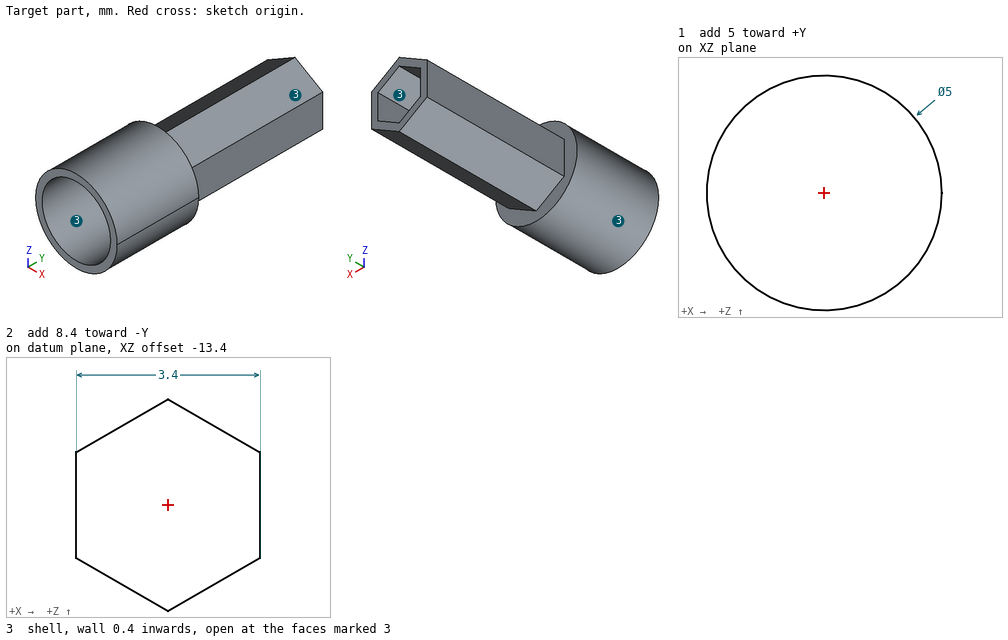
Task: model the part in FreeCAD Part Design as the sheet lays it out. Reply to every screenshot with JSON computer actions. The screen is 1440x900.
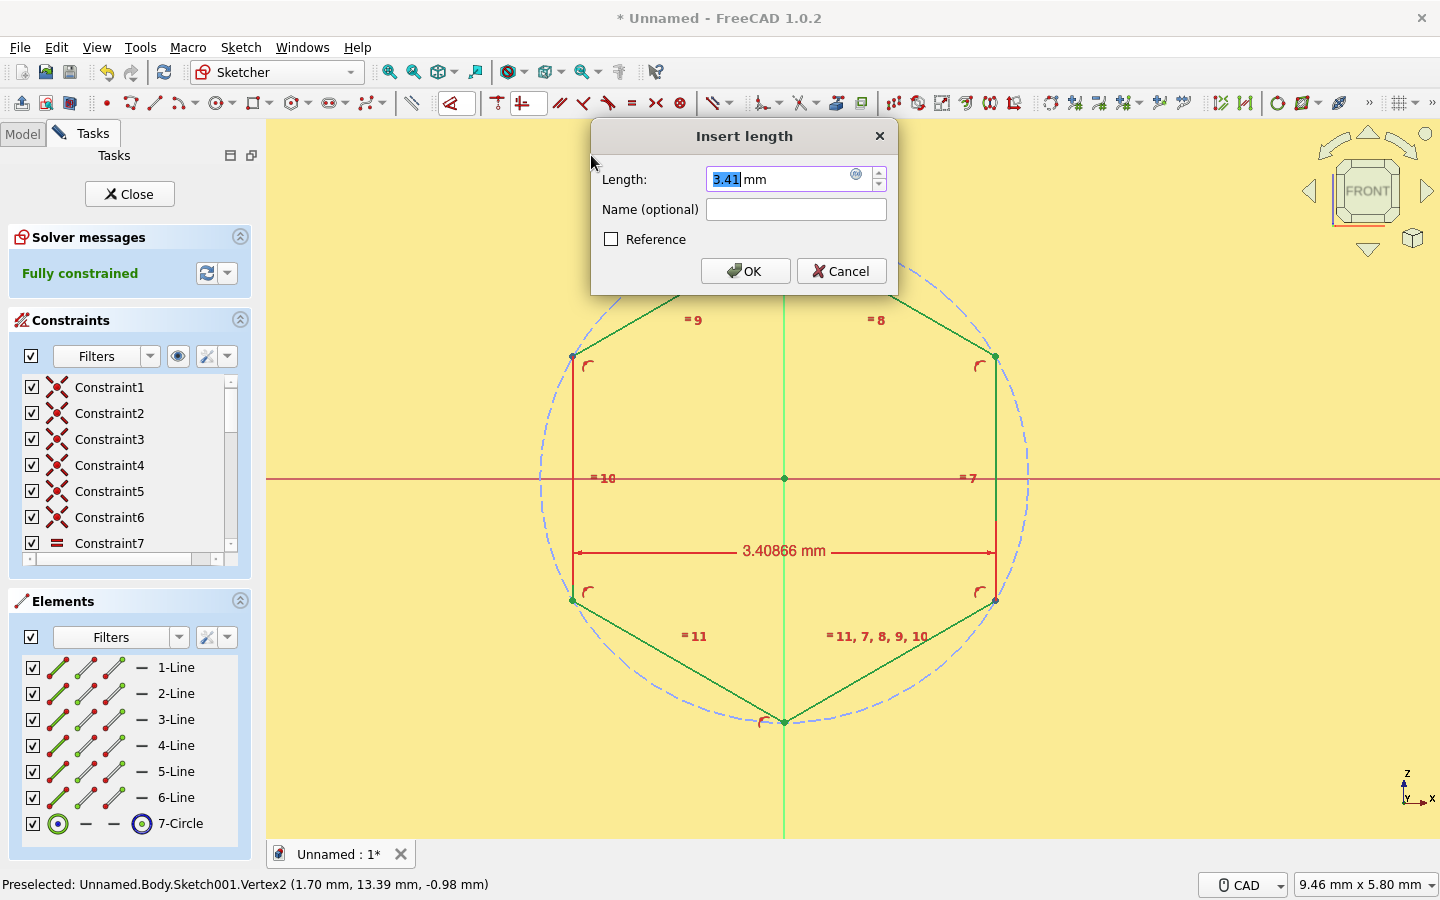
{"action": "type", "text": "3.4"}
{"action": "key", "text": "Return"}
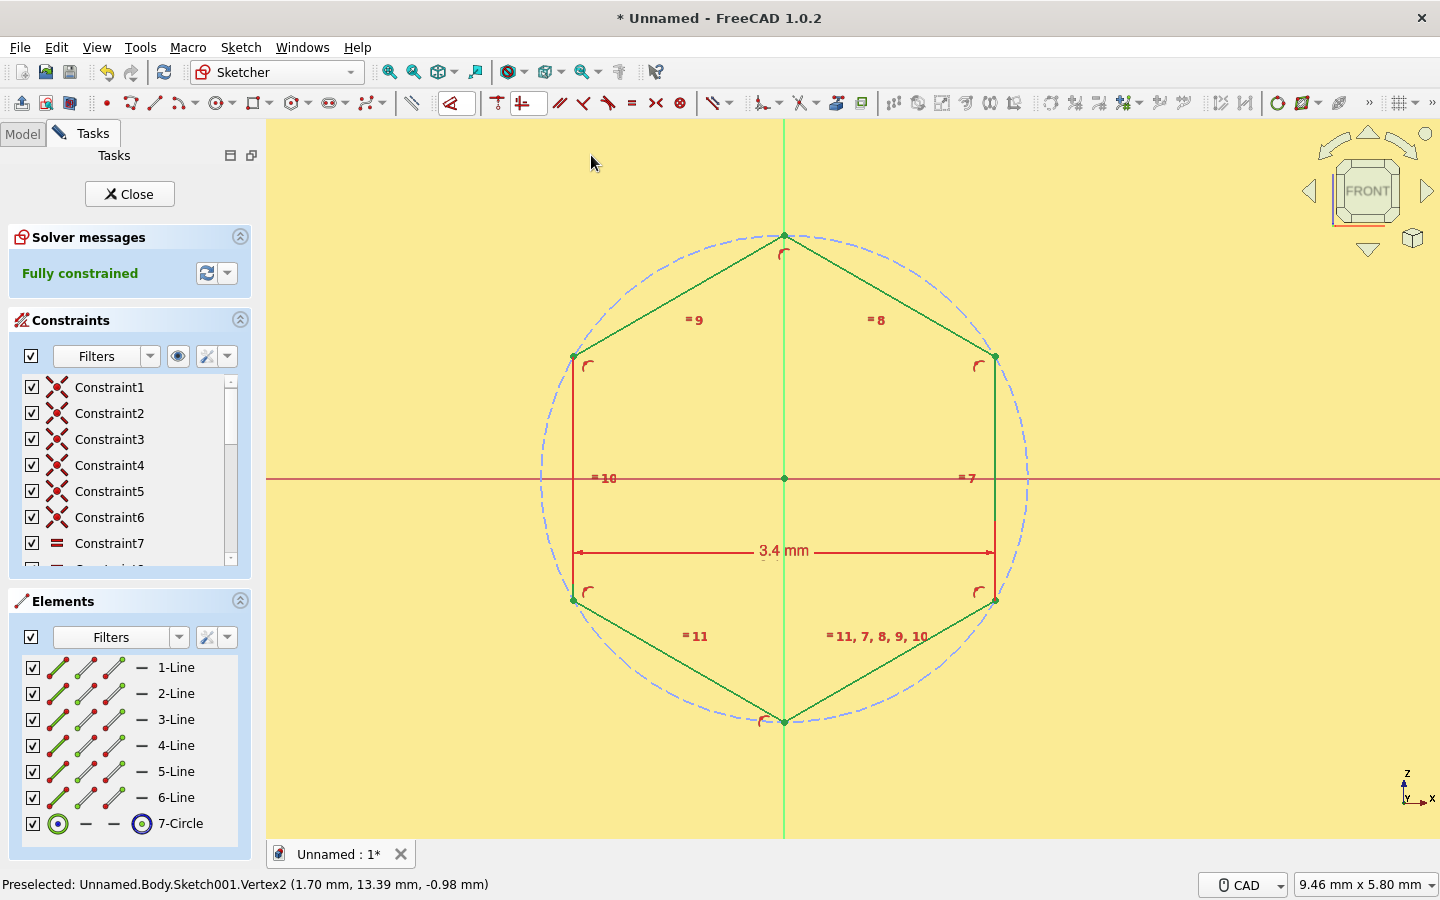
{"action": "left_click", "coordinate": [130, 194]}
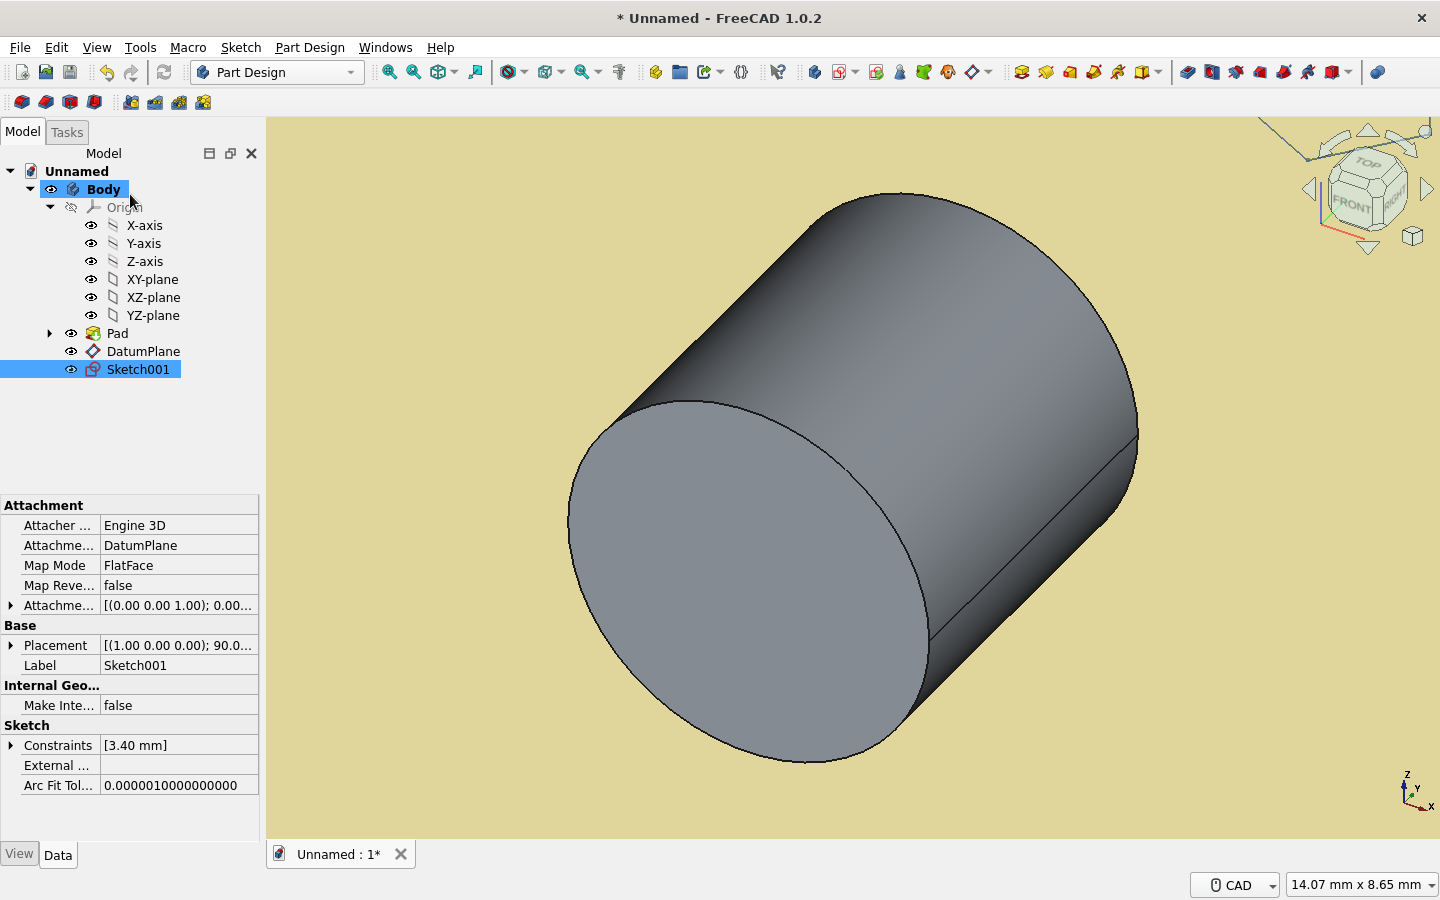
{"action": "left_click", "coordinate": [1022, 72]}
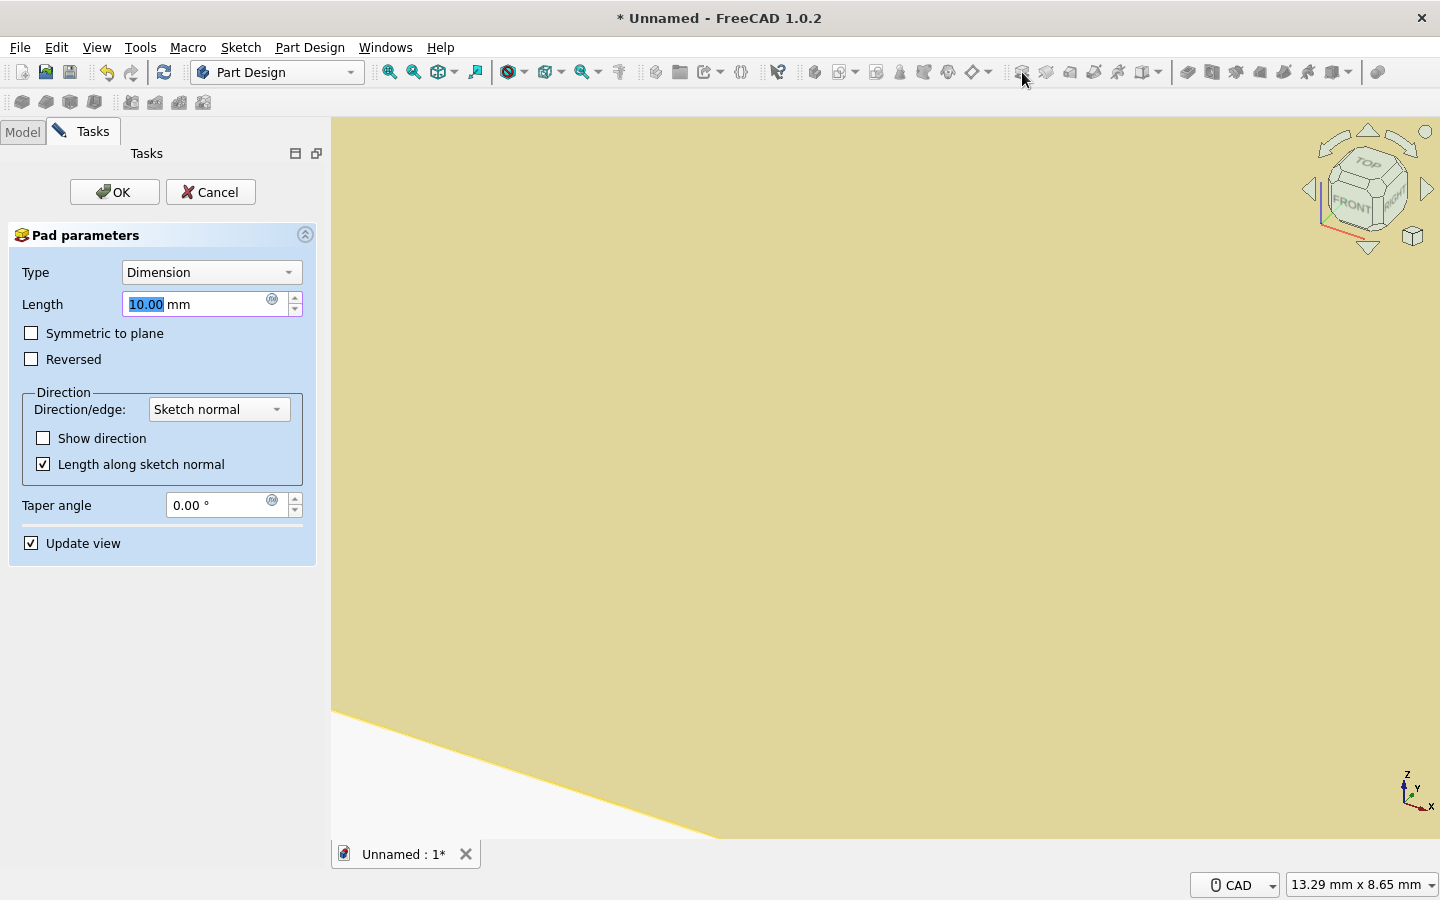
{"action": "type", "text": "8.4"}
{"action": "key", "text": "Tab"}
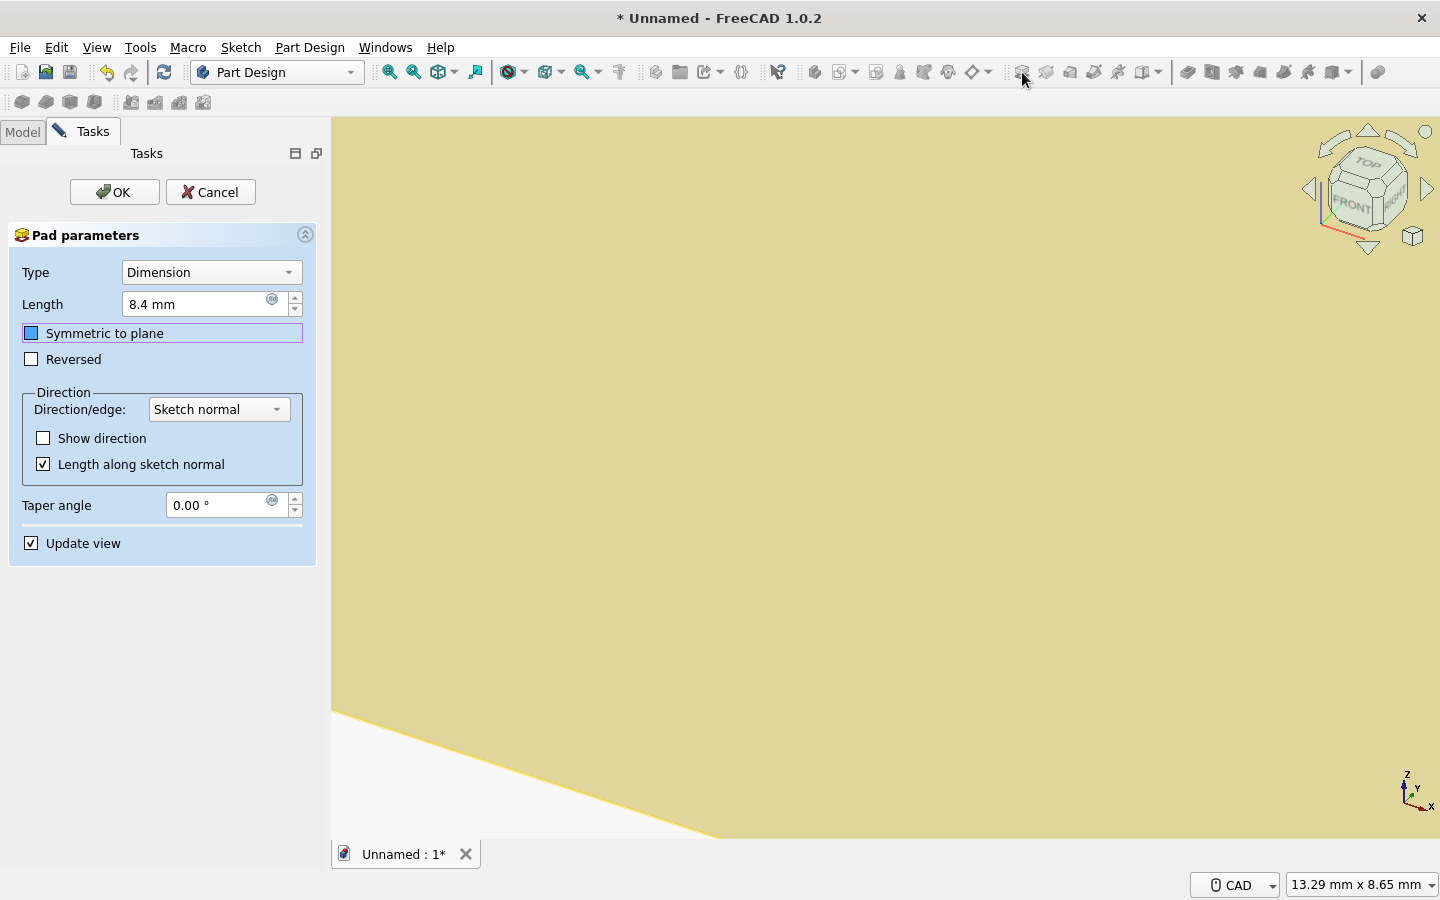
{"action": "left_click", "coordinate": [115, 192]}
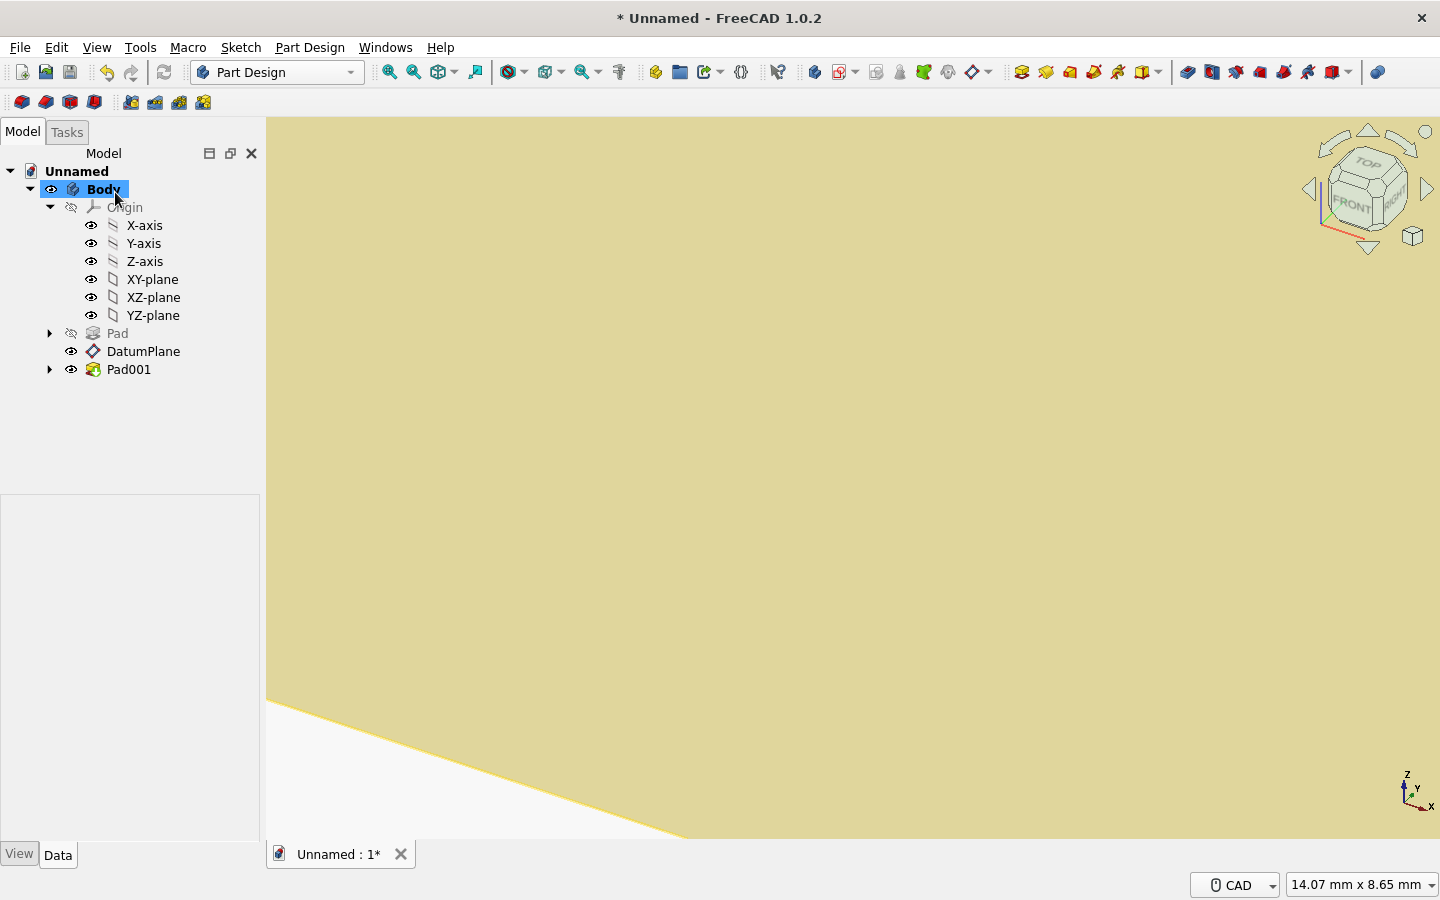
{"action": "left_click", "coordinate": [116, 351]}
{"action": "key", "text": "space"}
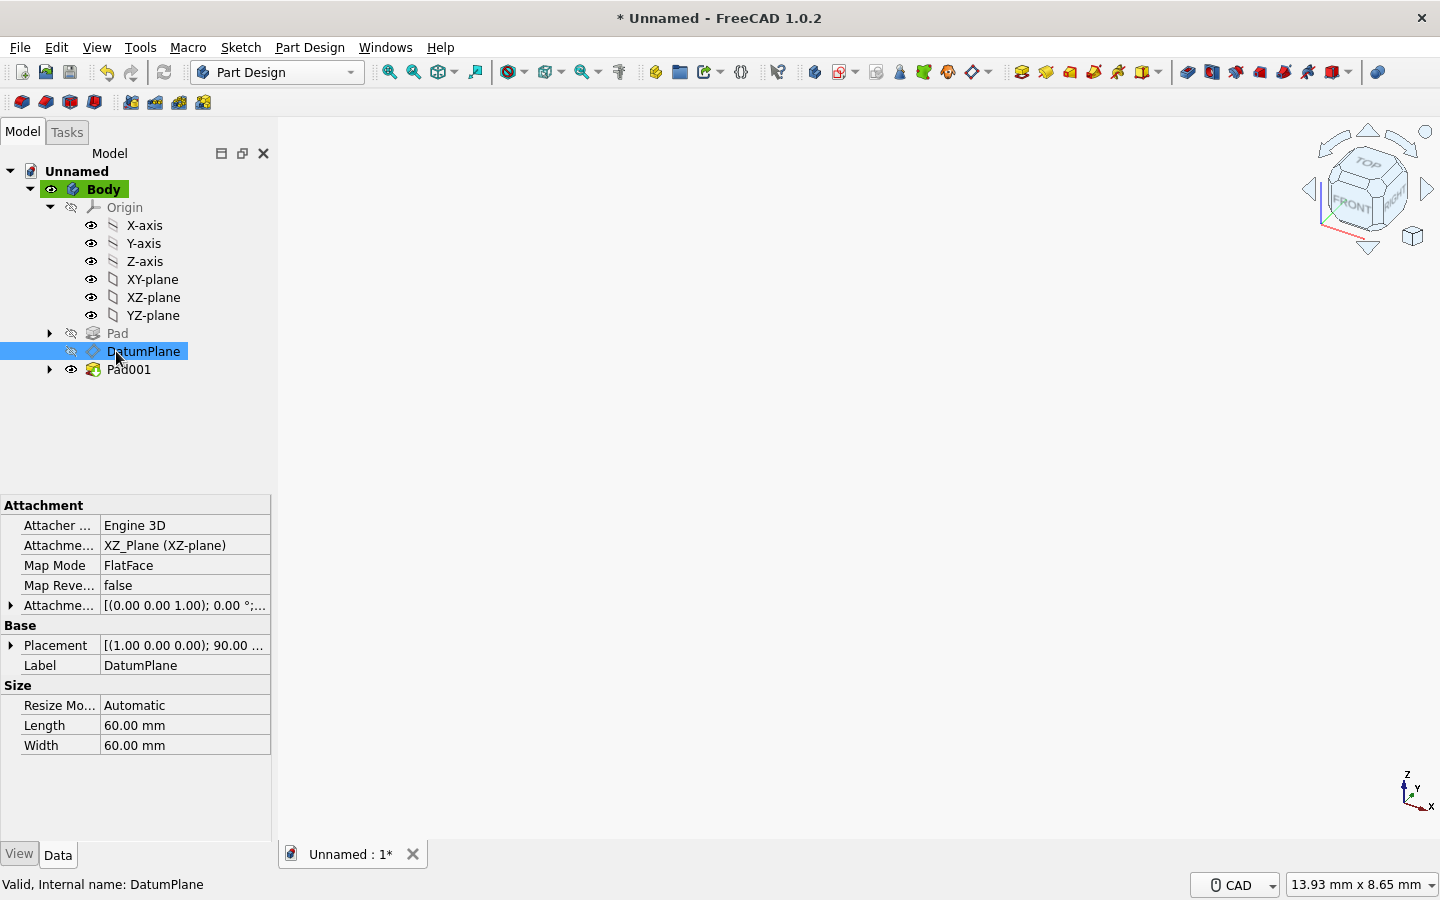
{"action": "left_click", "coordinate": [390, 72]}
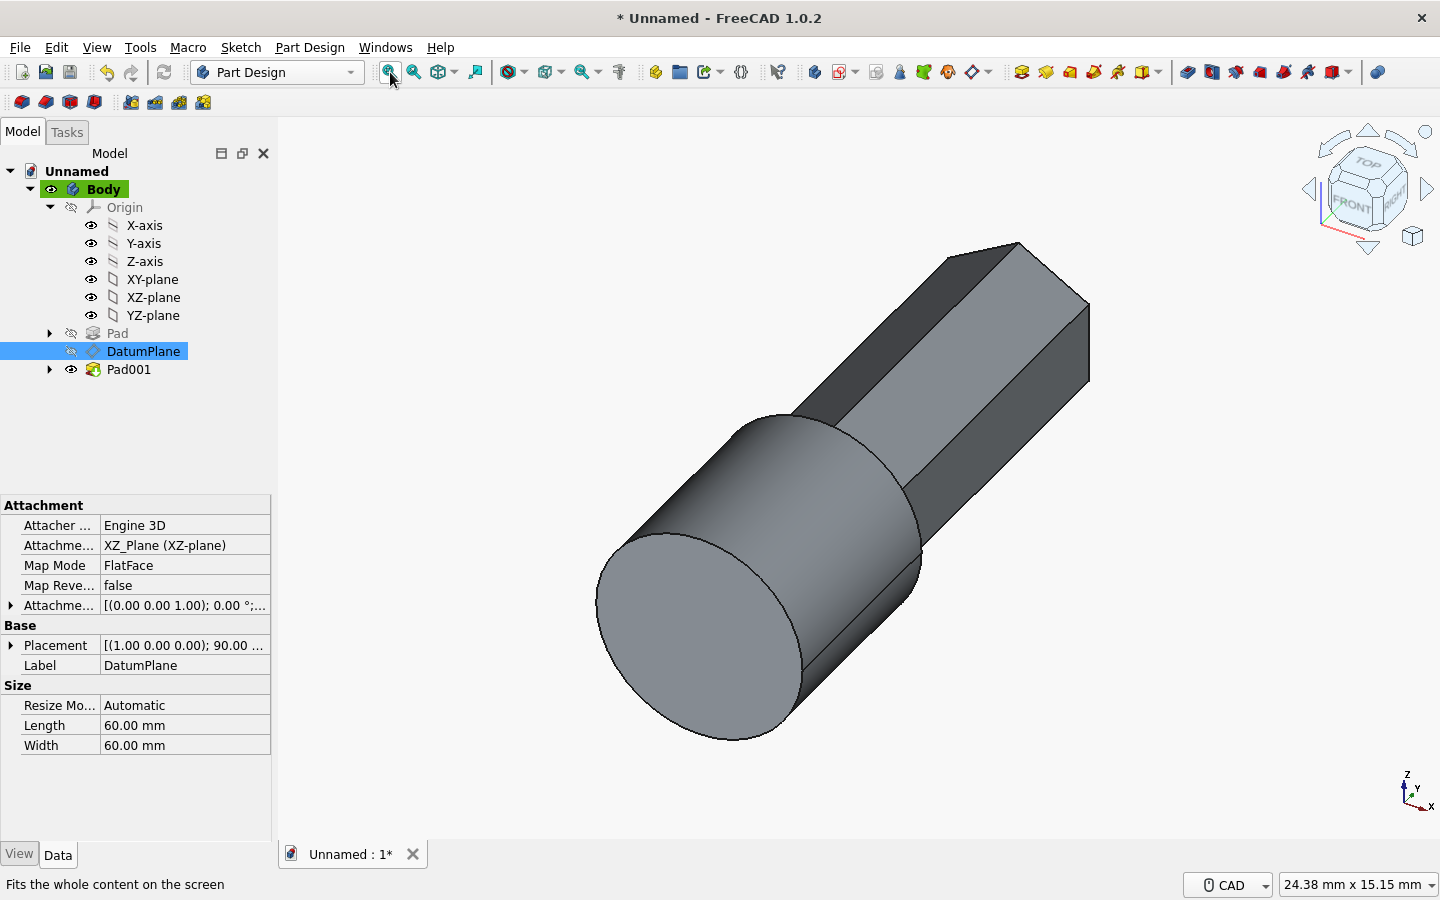
{"action": "left_click", "coordinate": [699, 636]}